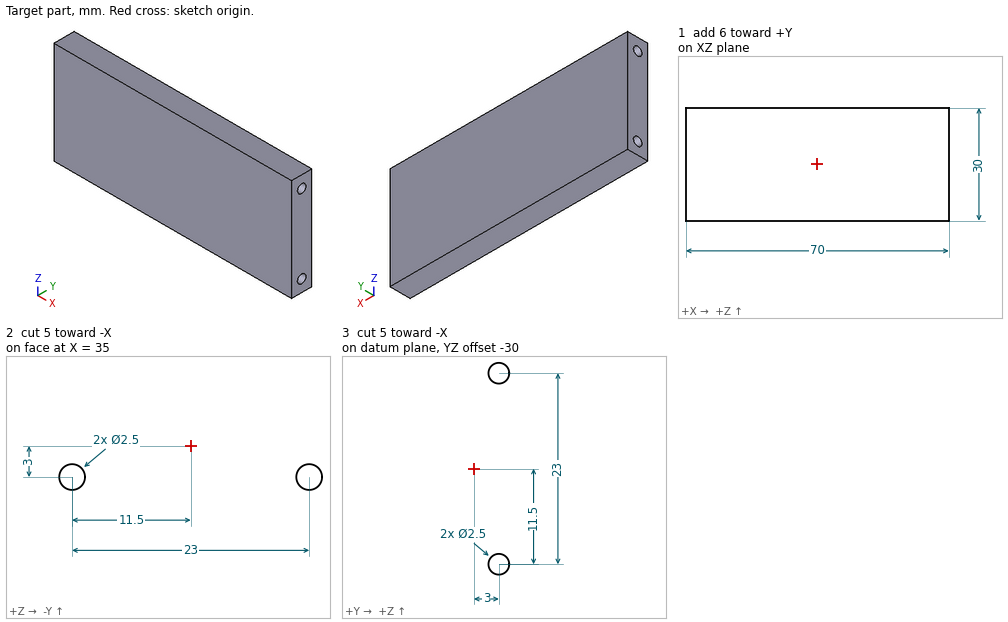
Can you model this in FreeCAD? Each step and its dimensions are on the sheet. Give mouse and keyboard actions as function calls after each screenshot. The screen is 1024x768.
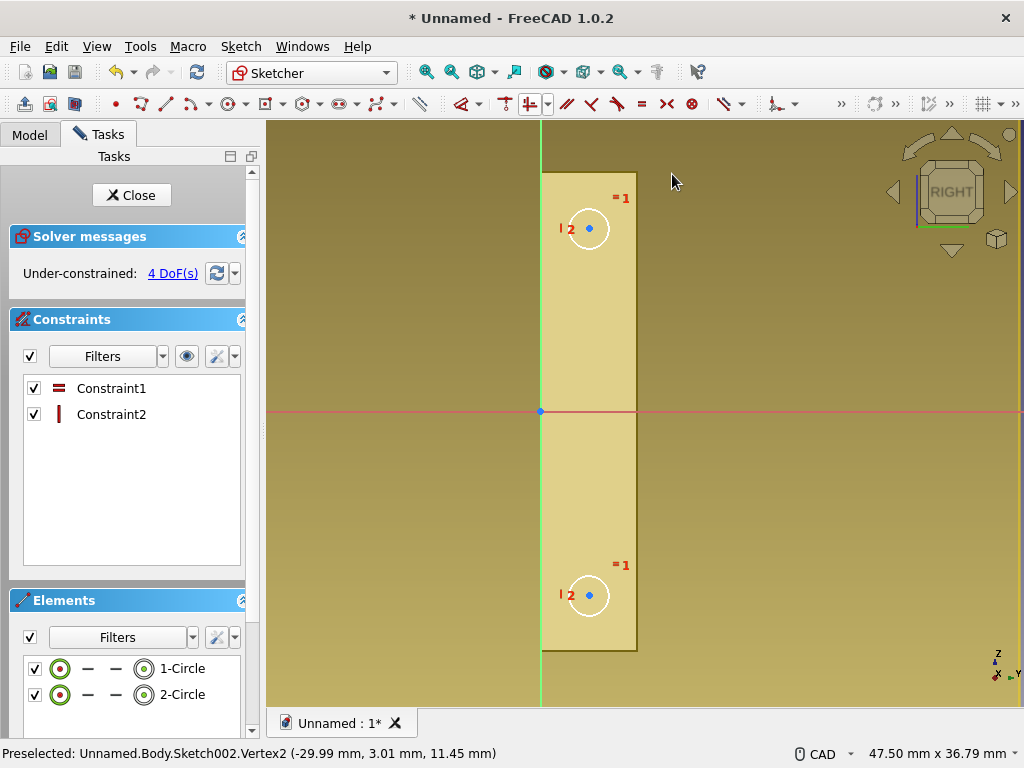
click(460, 104)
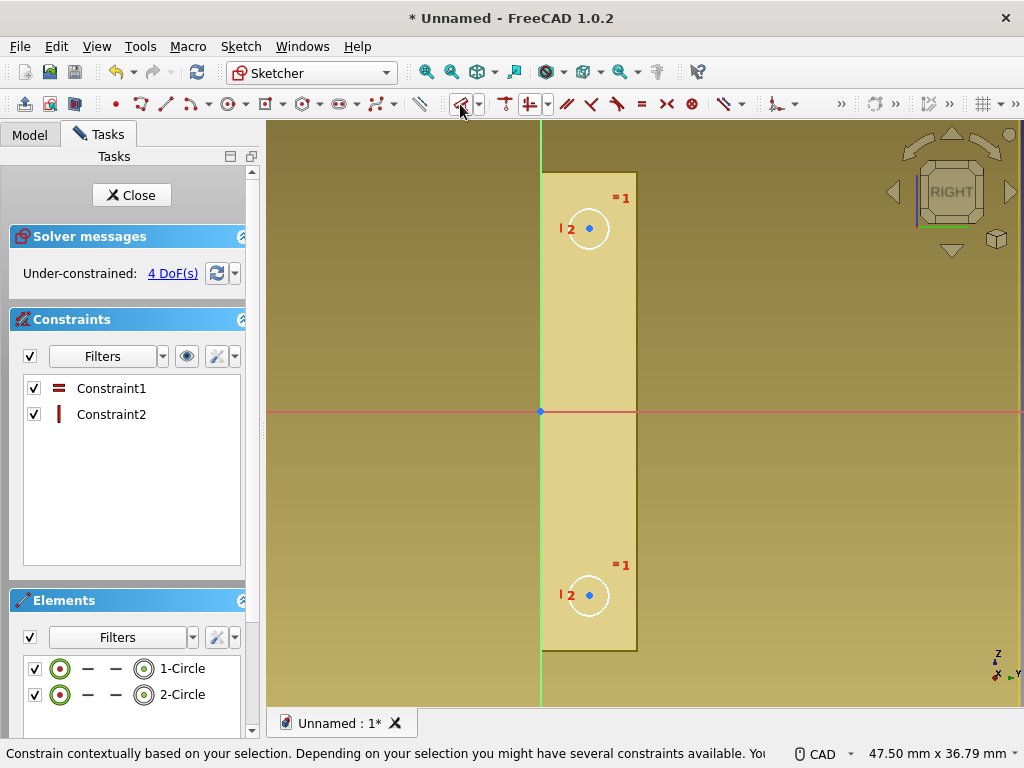
click(603, 582)
click(626, 559)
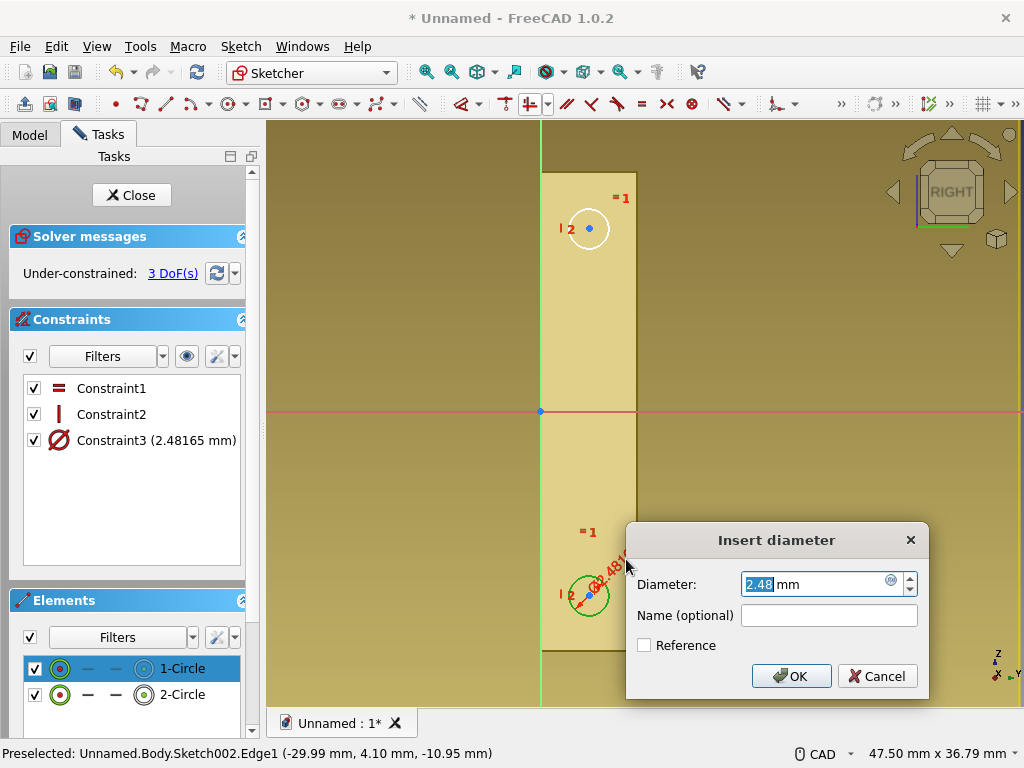
text(2.5)
key(Return)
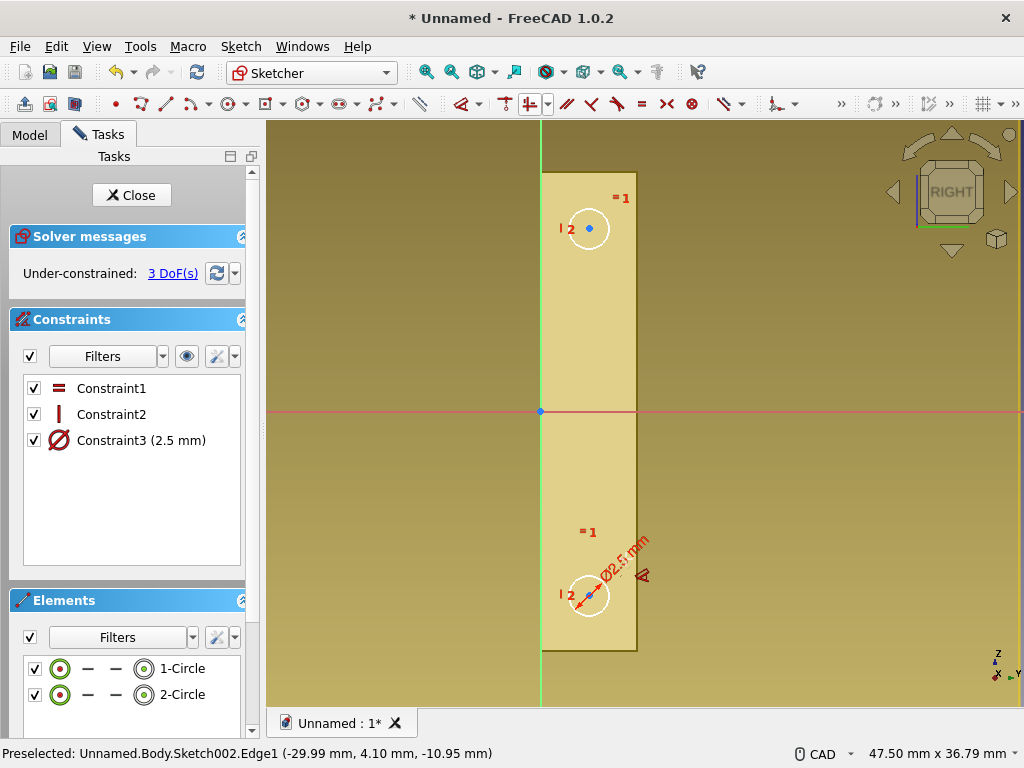
click(589, 596)
click(565, 630)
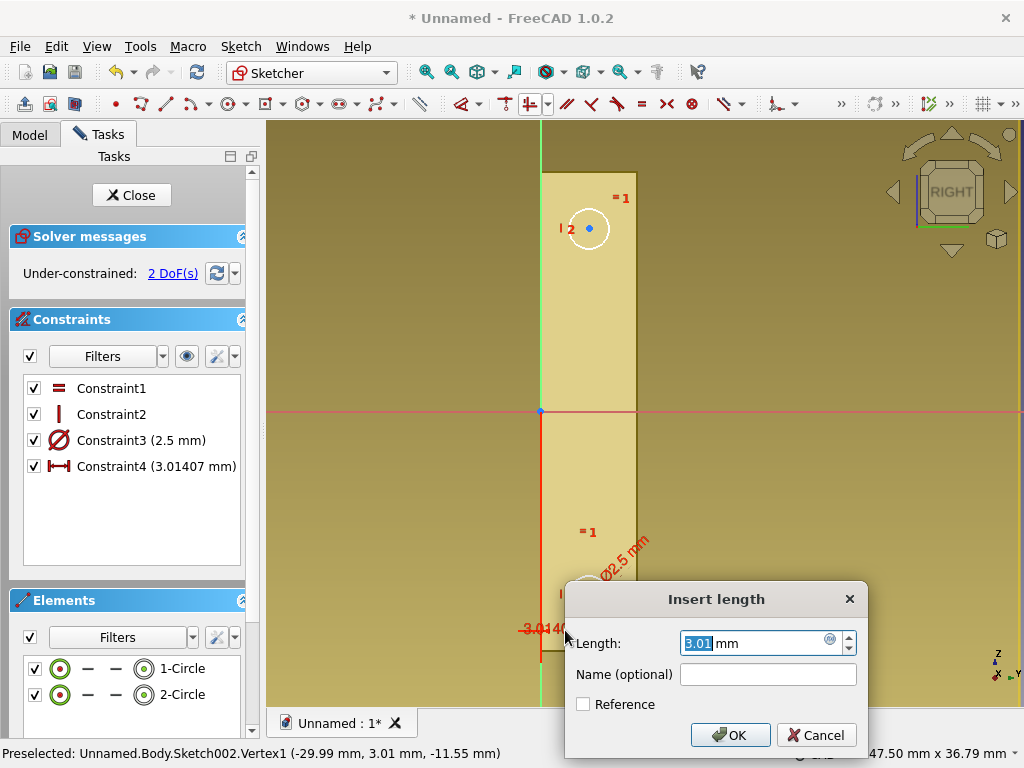
text(3)
key(Return)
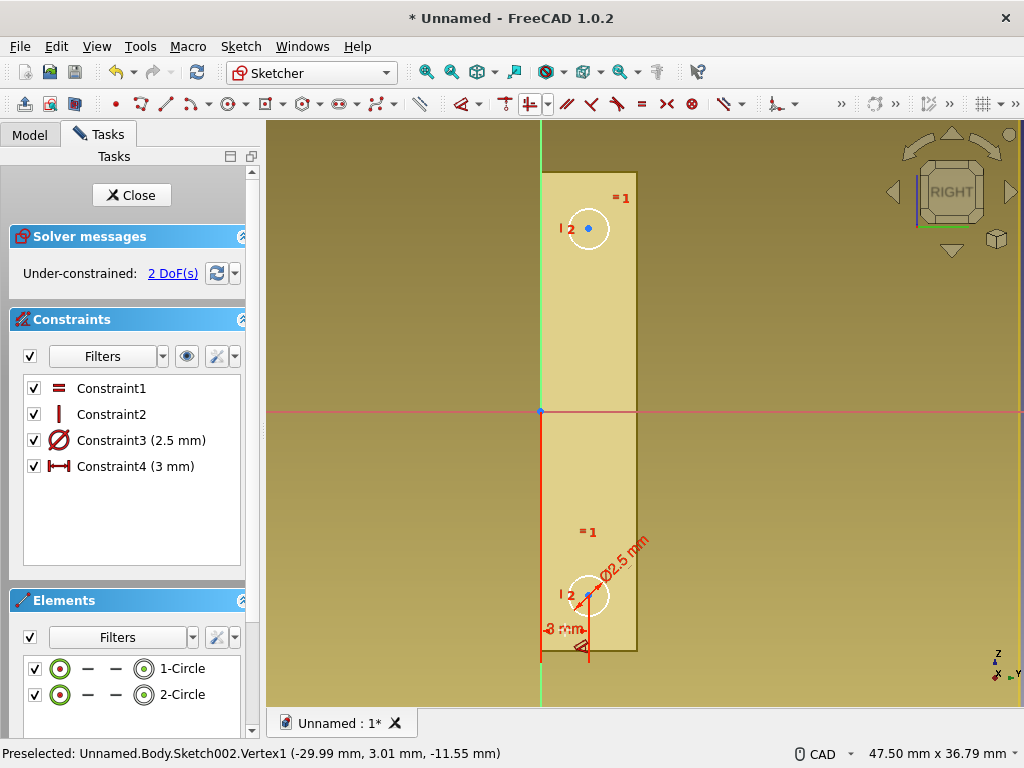
click(589, 596)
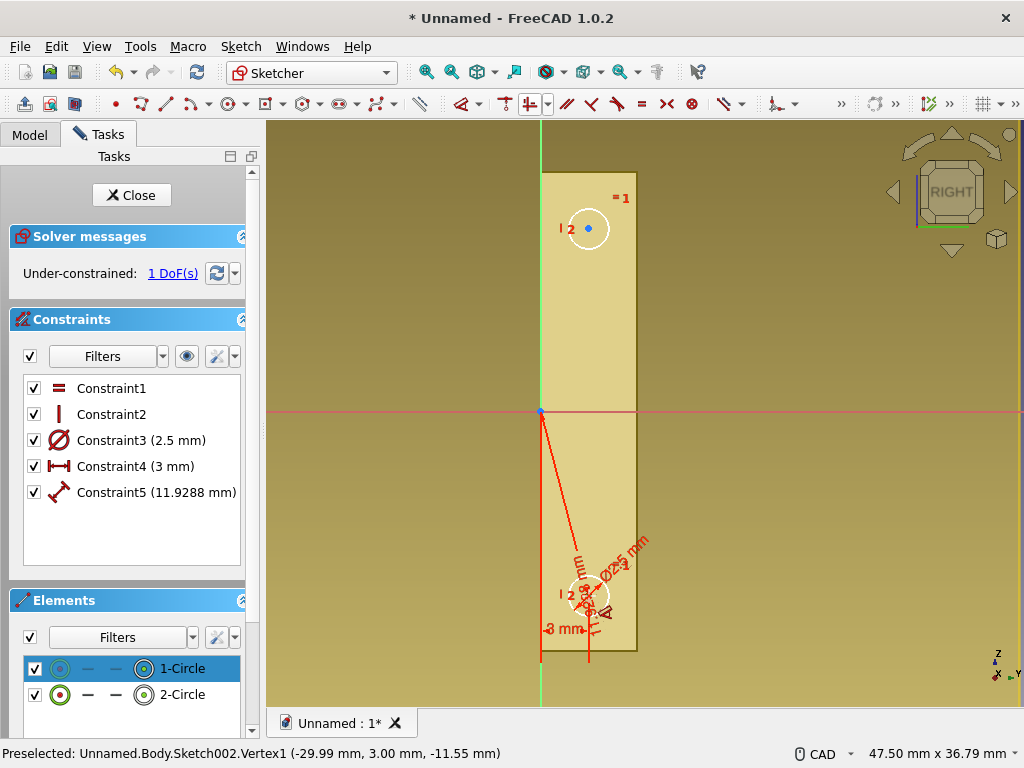
click(589, 229)
click(623, 328)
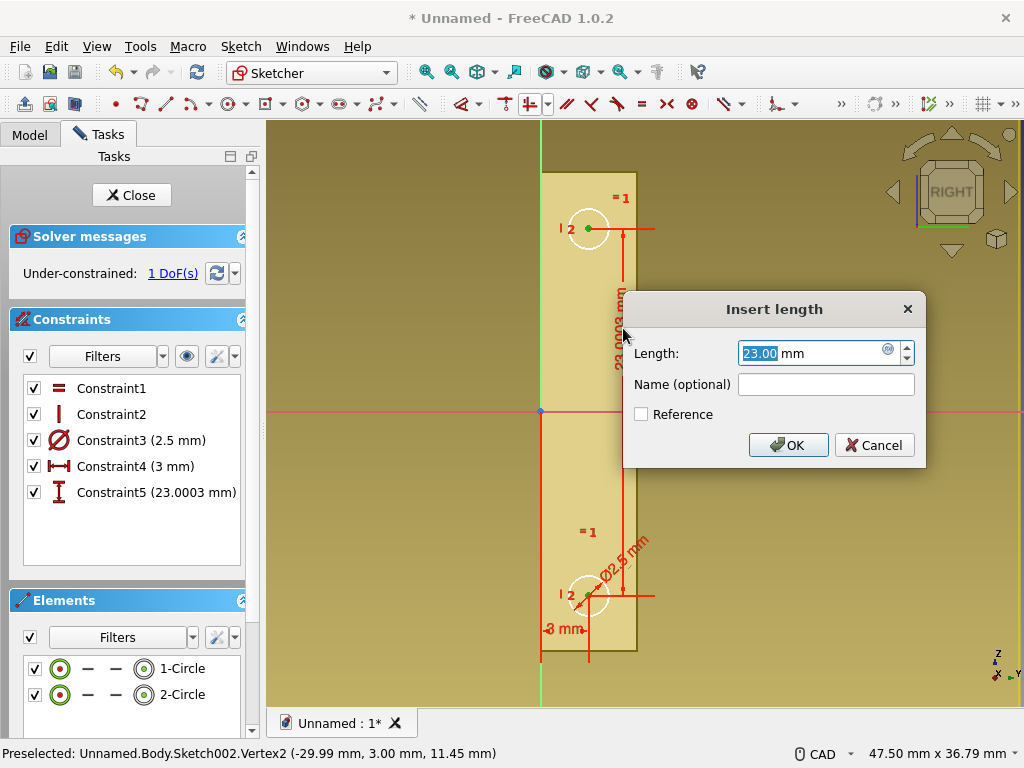
text(23)
key(Return)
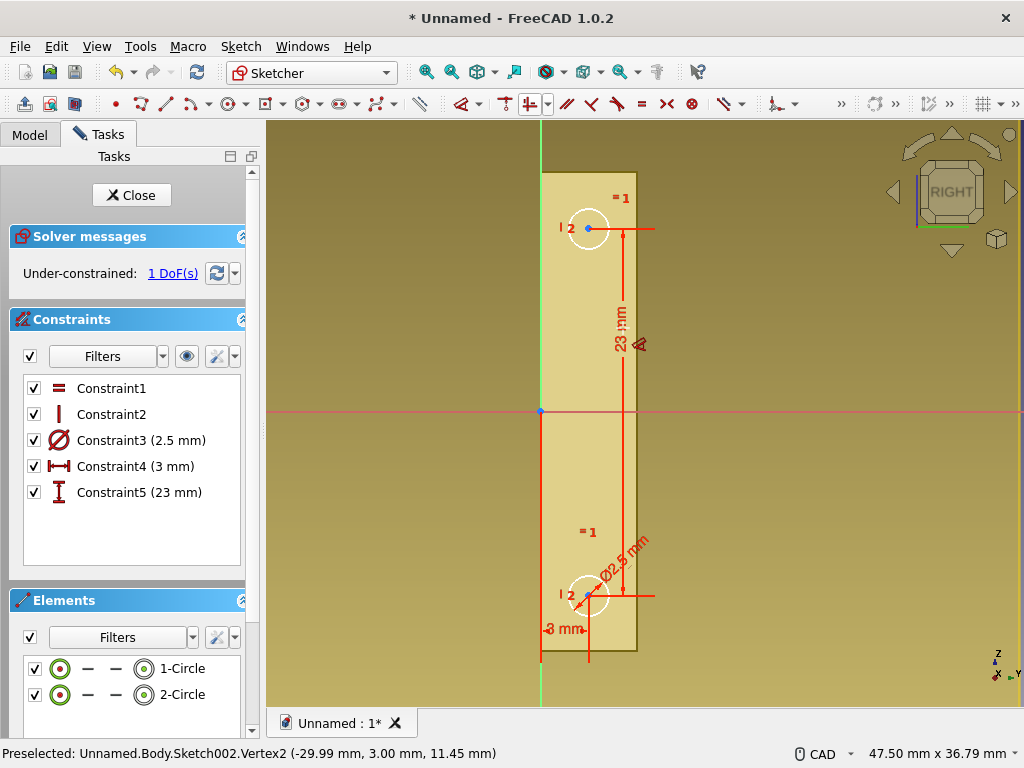
click(589, 596)
click(507, 504)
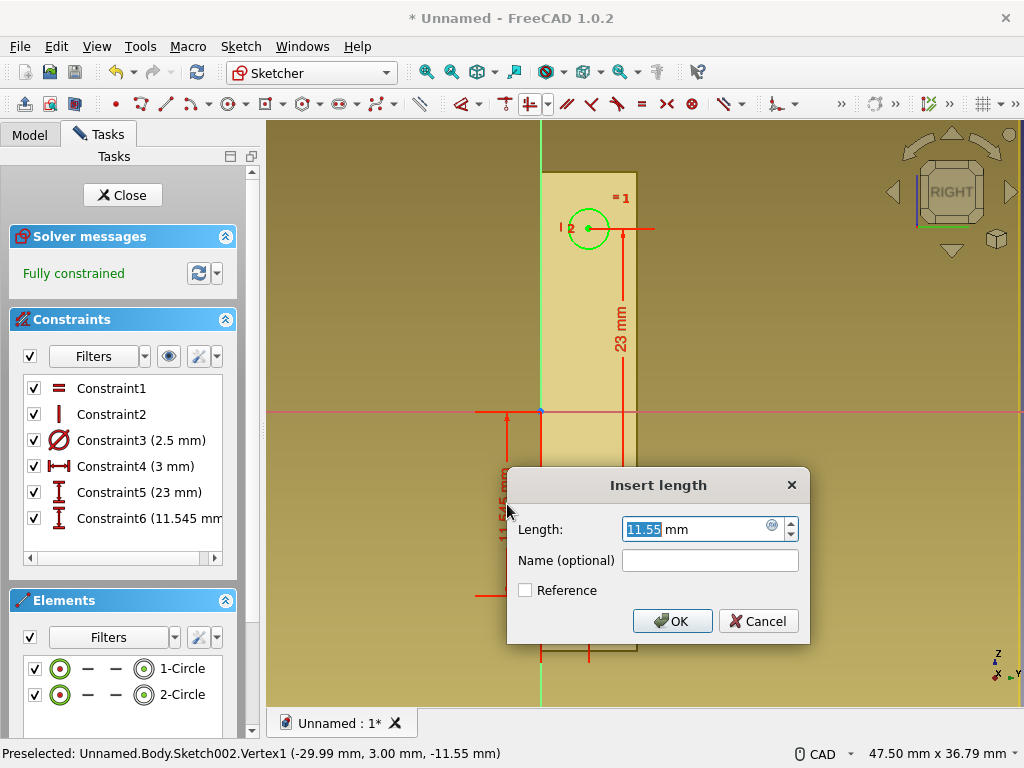
text(11.5)
key(Return)
key(Escape)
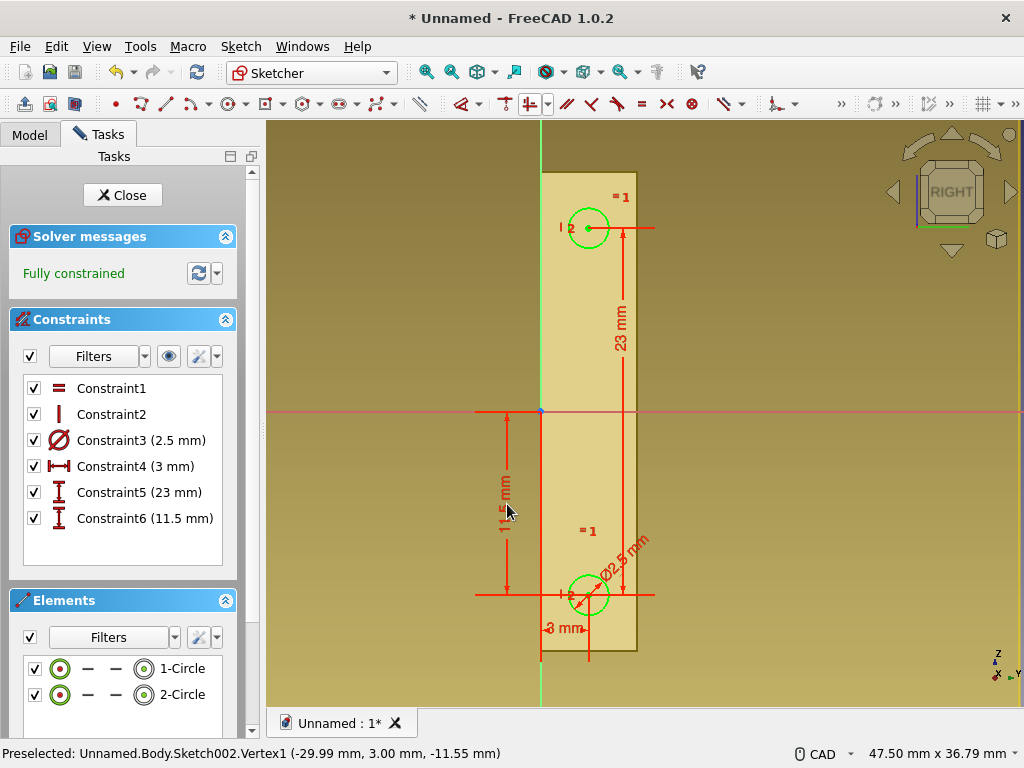
click(123, 195)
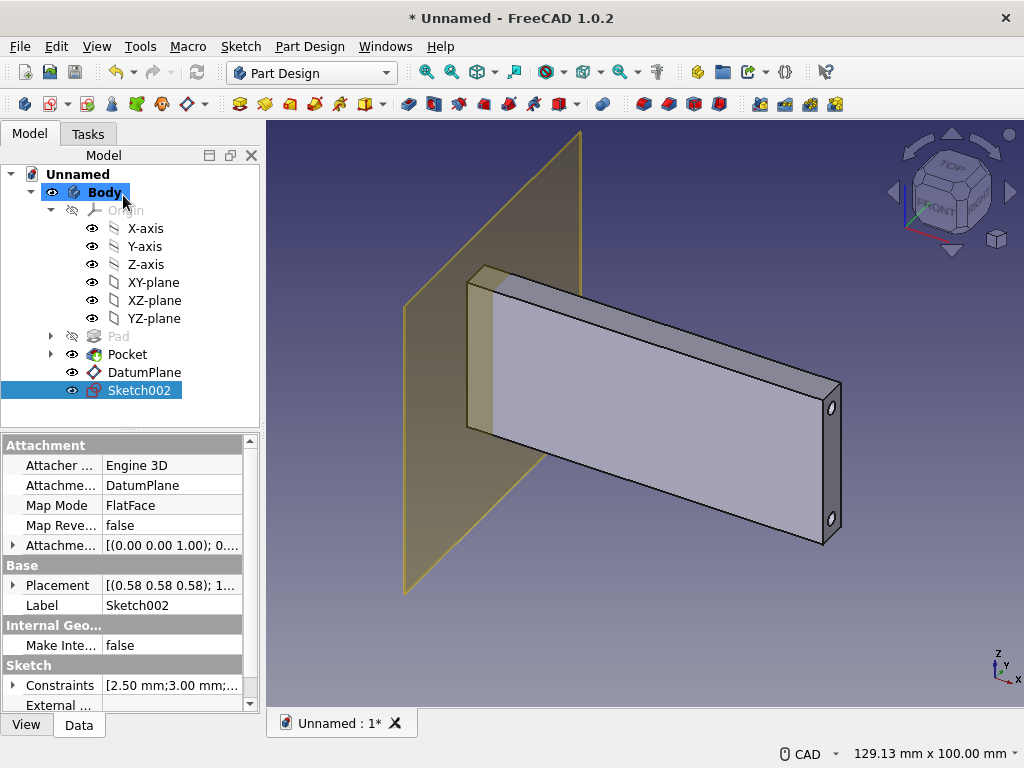
click(409, 104)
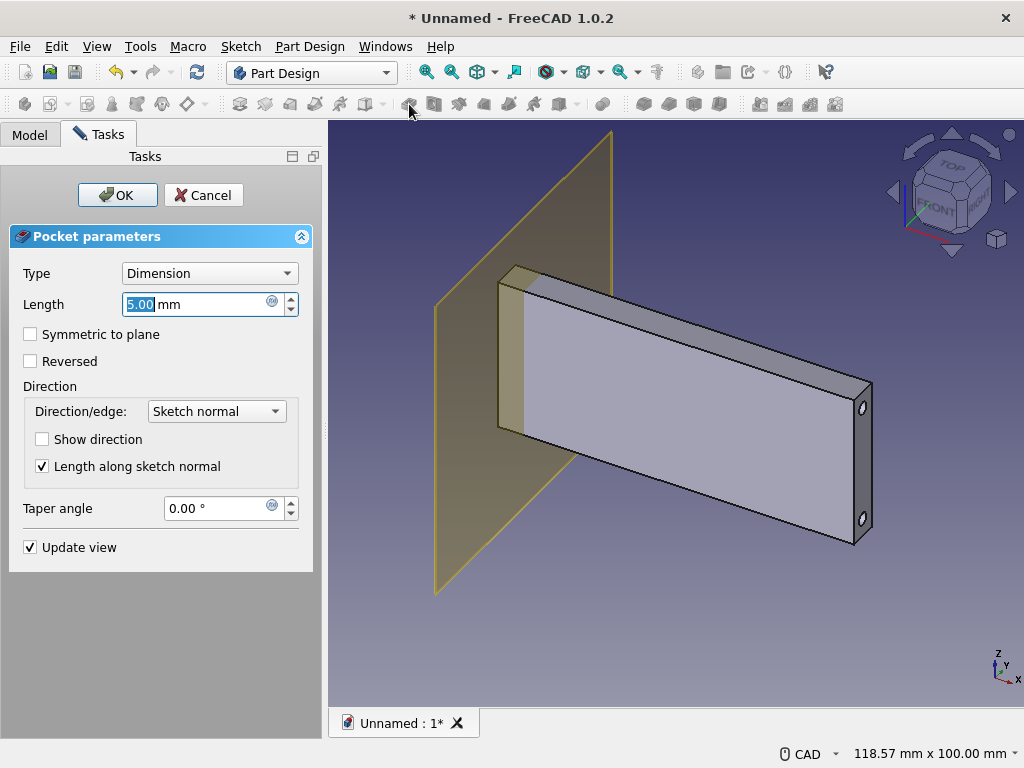
text(5)
key(Tab)